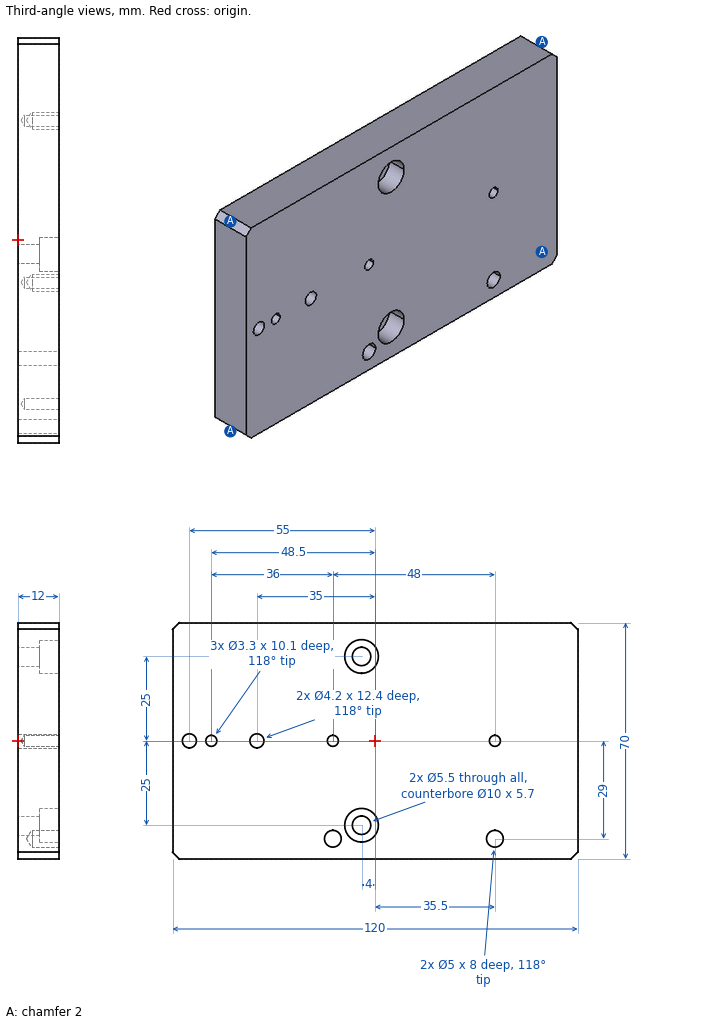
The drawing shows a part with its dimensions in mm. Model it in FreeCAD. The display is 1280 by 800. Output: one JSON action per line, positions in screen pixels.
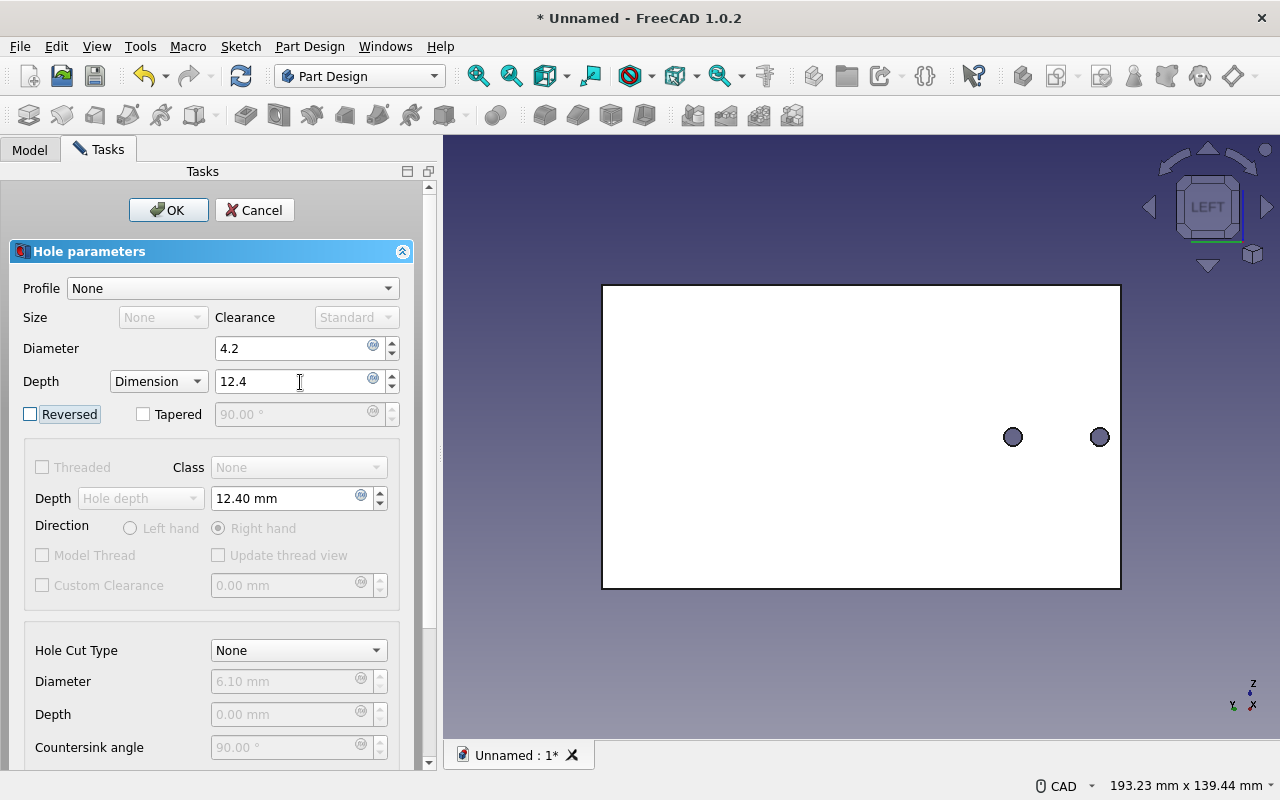
{"action": "left_click", "coordinate": [169, 210]}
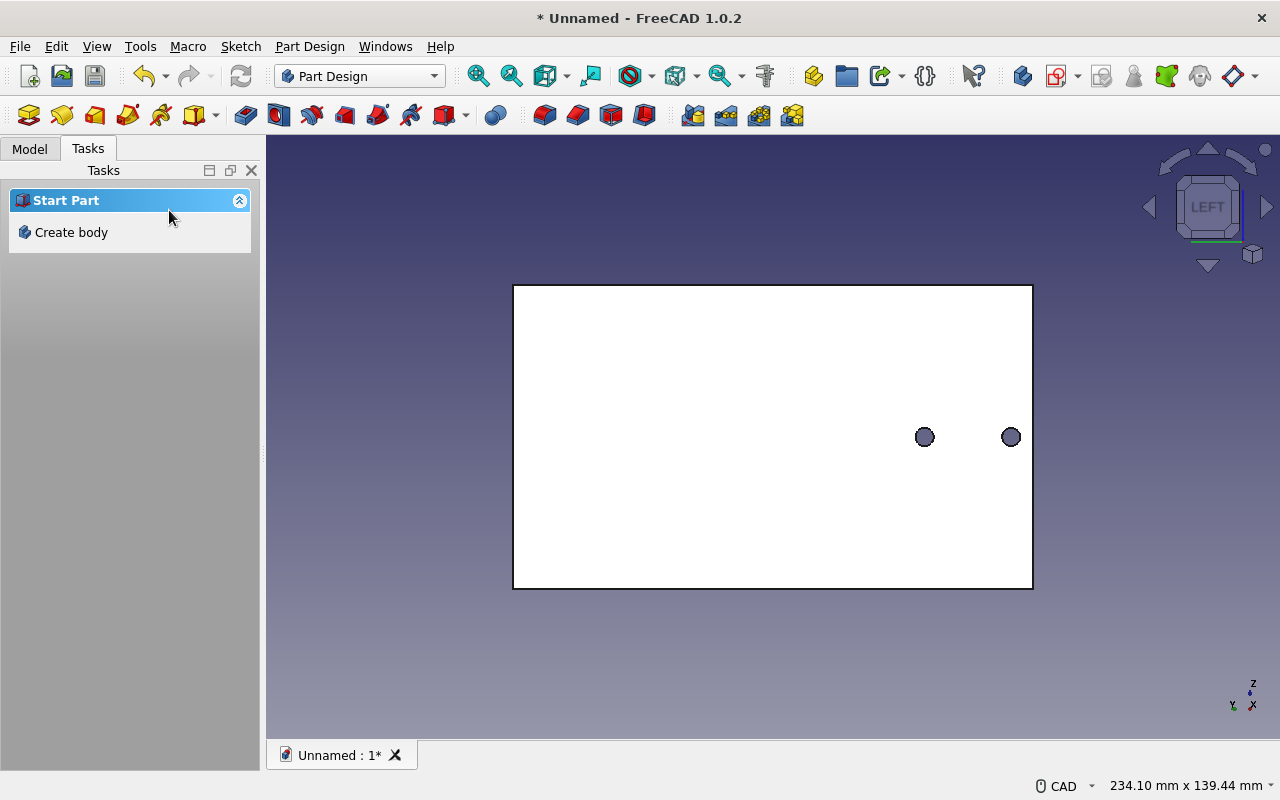
{"action": "key", "text": "0"}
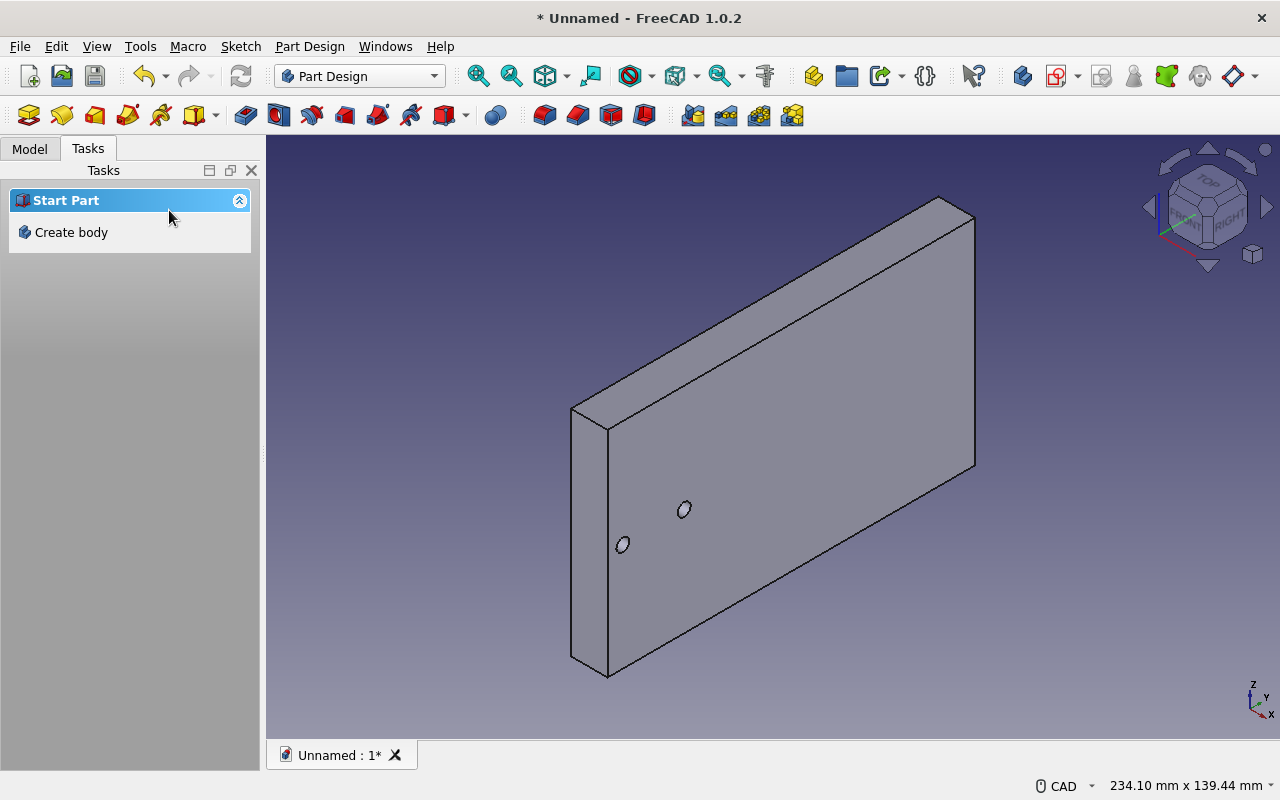
{"action": "left_click", "coordinate": [844, 416]}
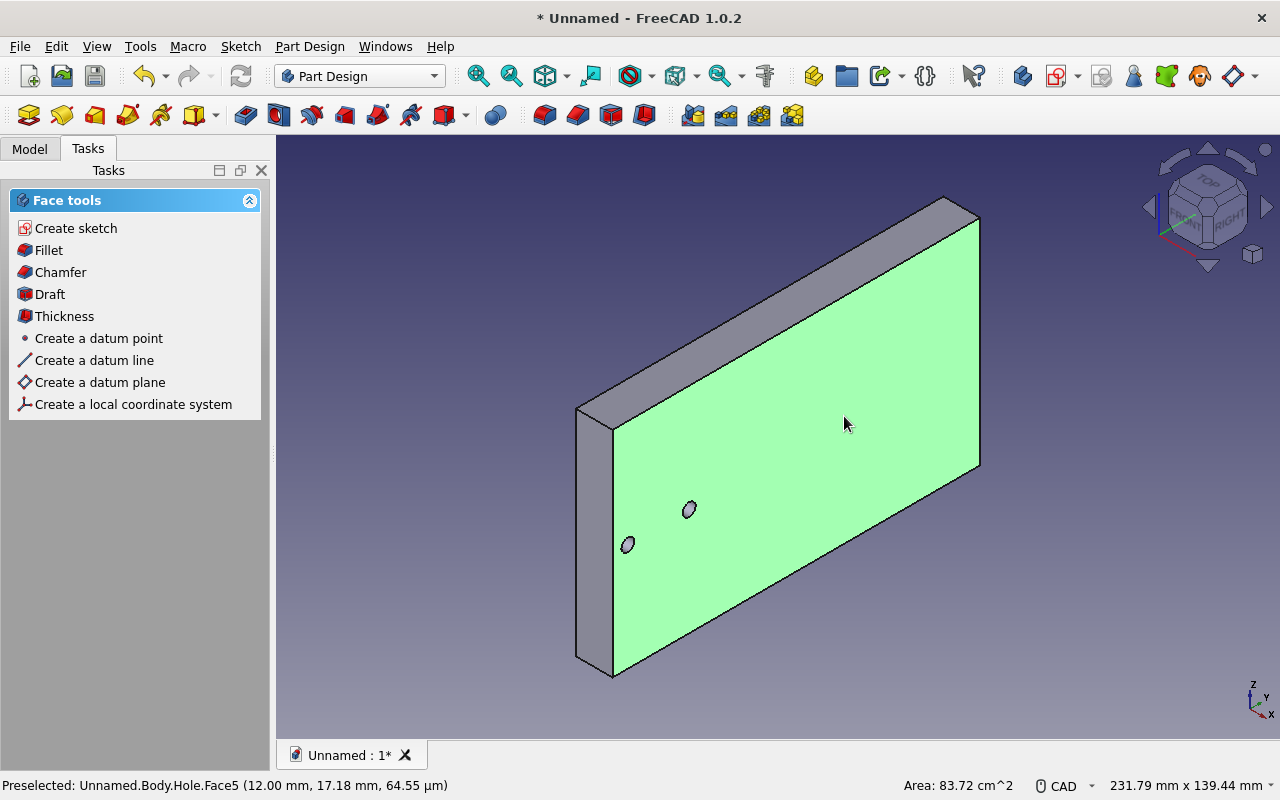
{"action": "left_click", "coordinate": [1056, 76]}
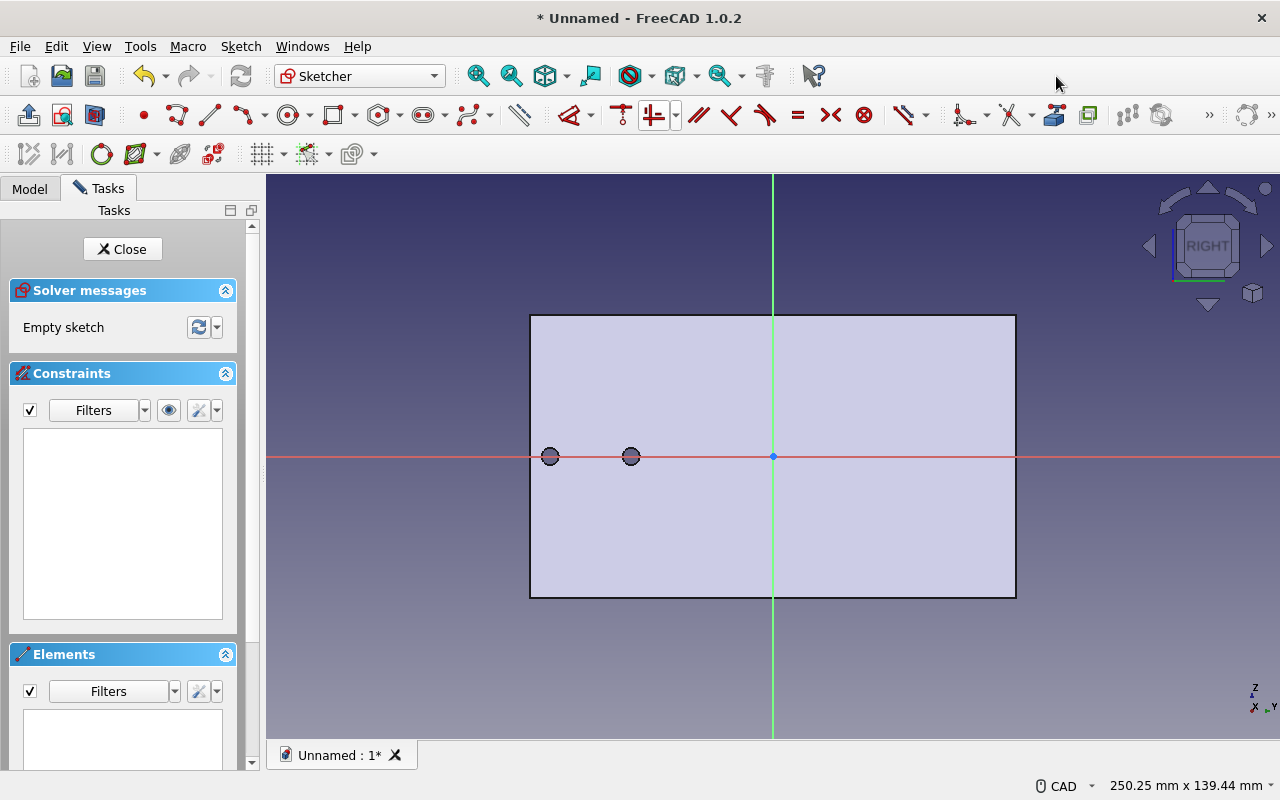
{"action": "scroll", "coordinate": [871, 457], "scroll_direction": "up", "scroll_amount": 2}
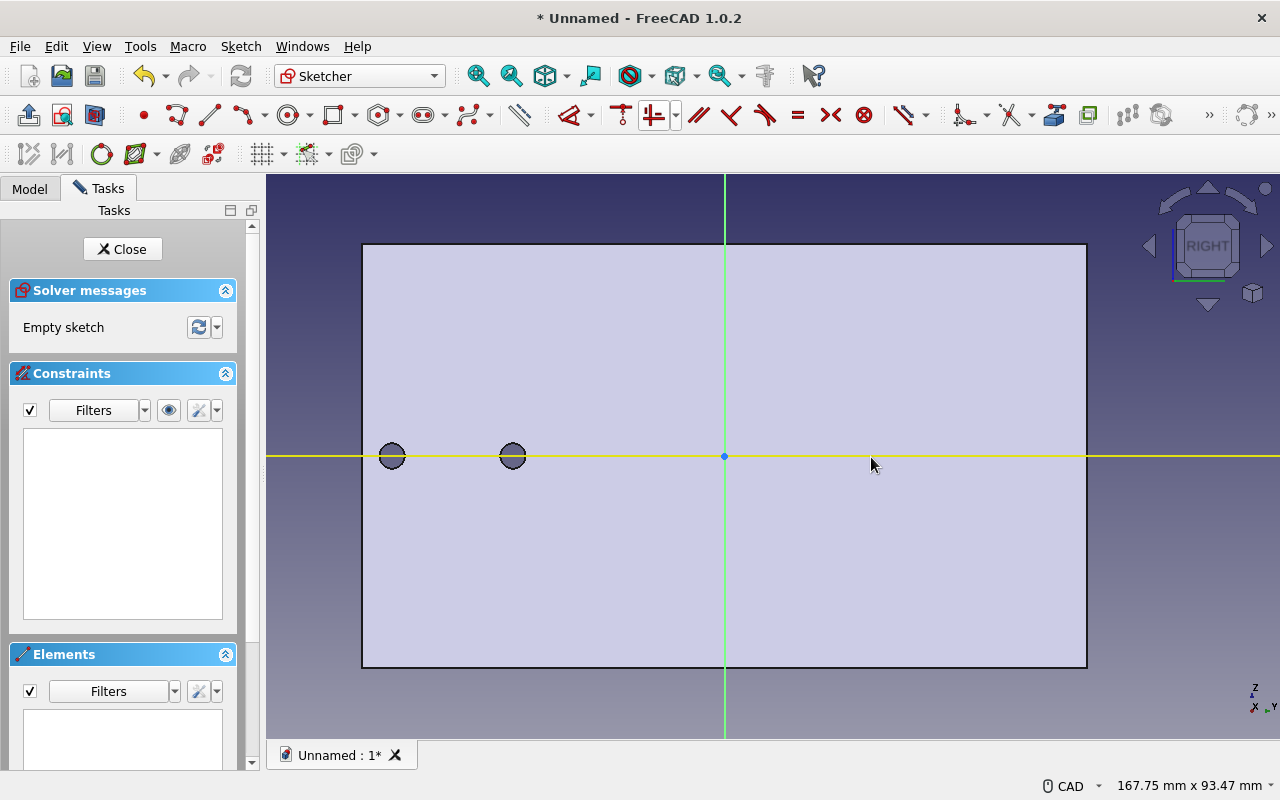
{"action": "left_click", "coordinate": [288, 116]}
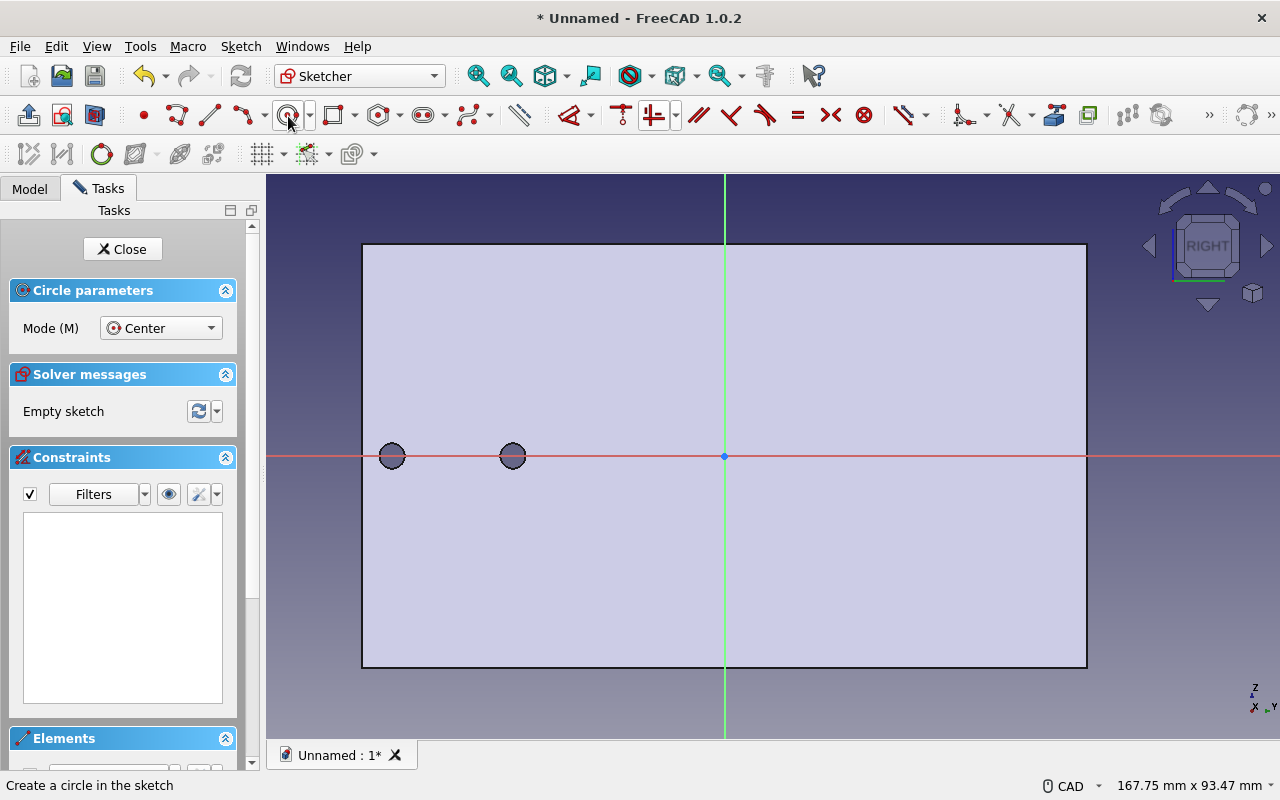
{"action": "scroll", "coordinate": [700, 607], "scroll_direction": "up", "scroll_amount": 2}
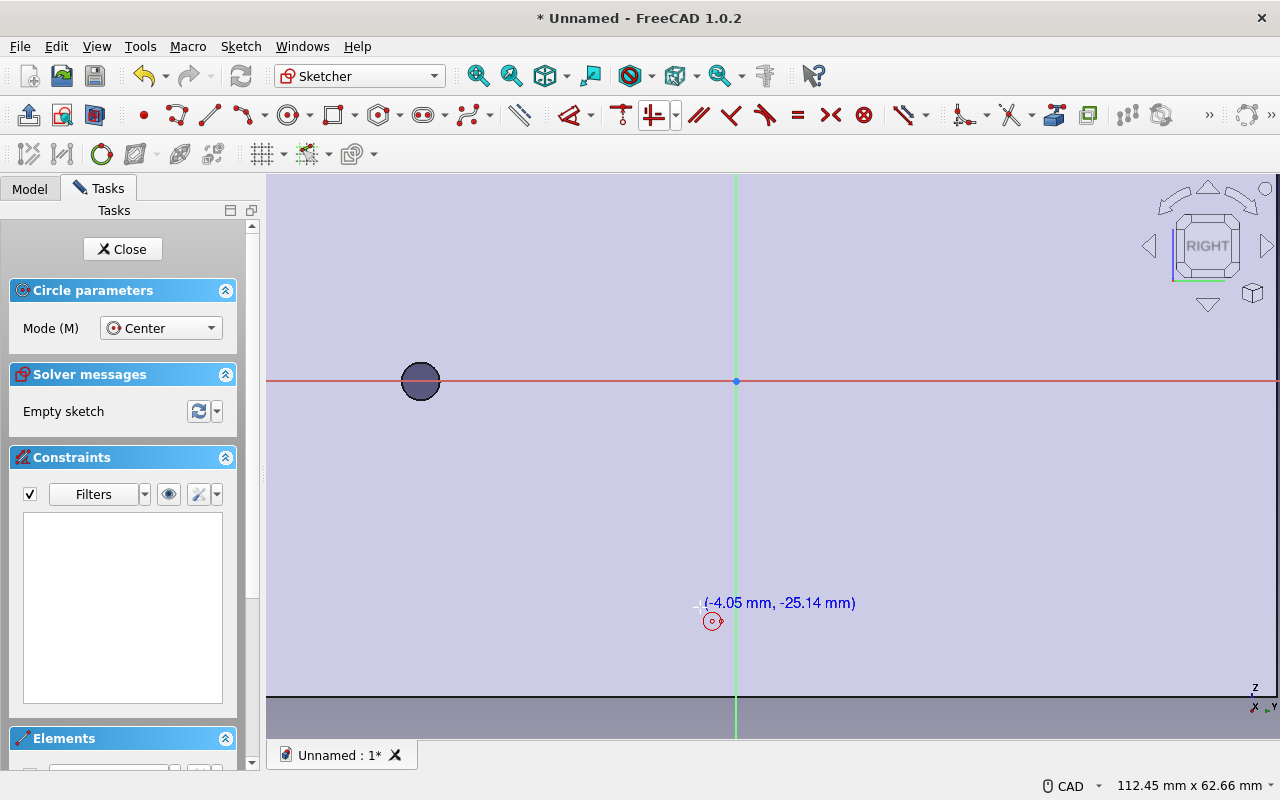
{"action": "left_click", "coordinate": [700, 607]}
{"action": "left_click", "coordinate": [718, 589]}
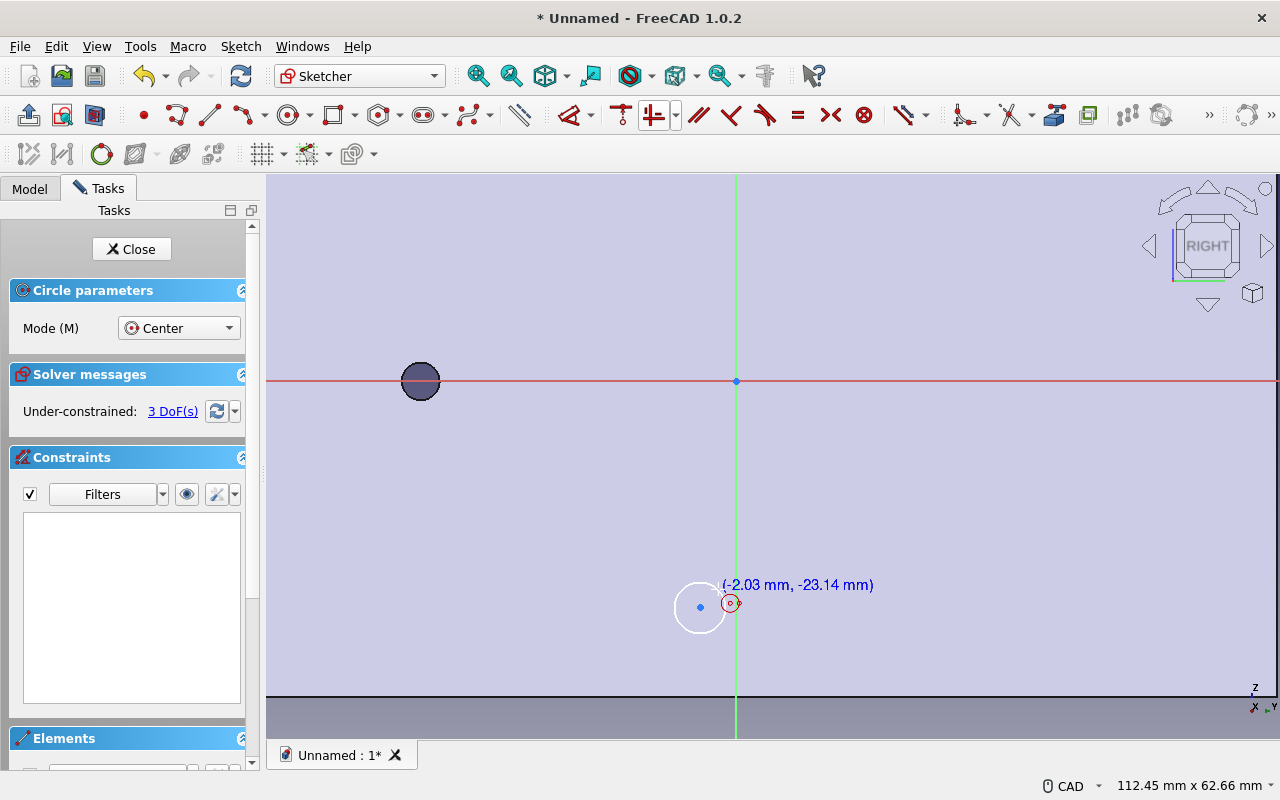
{"action": "scroll", "coordinate": [702, 609], "scroll_direction": "down", "scroll_amount": 2}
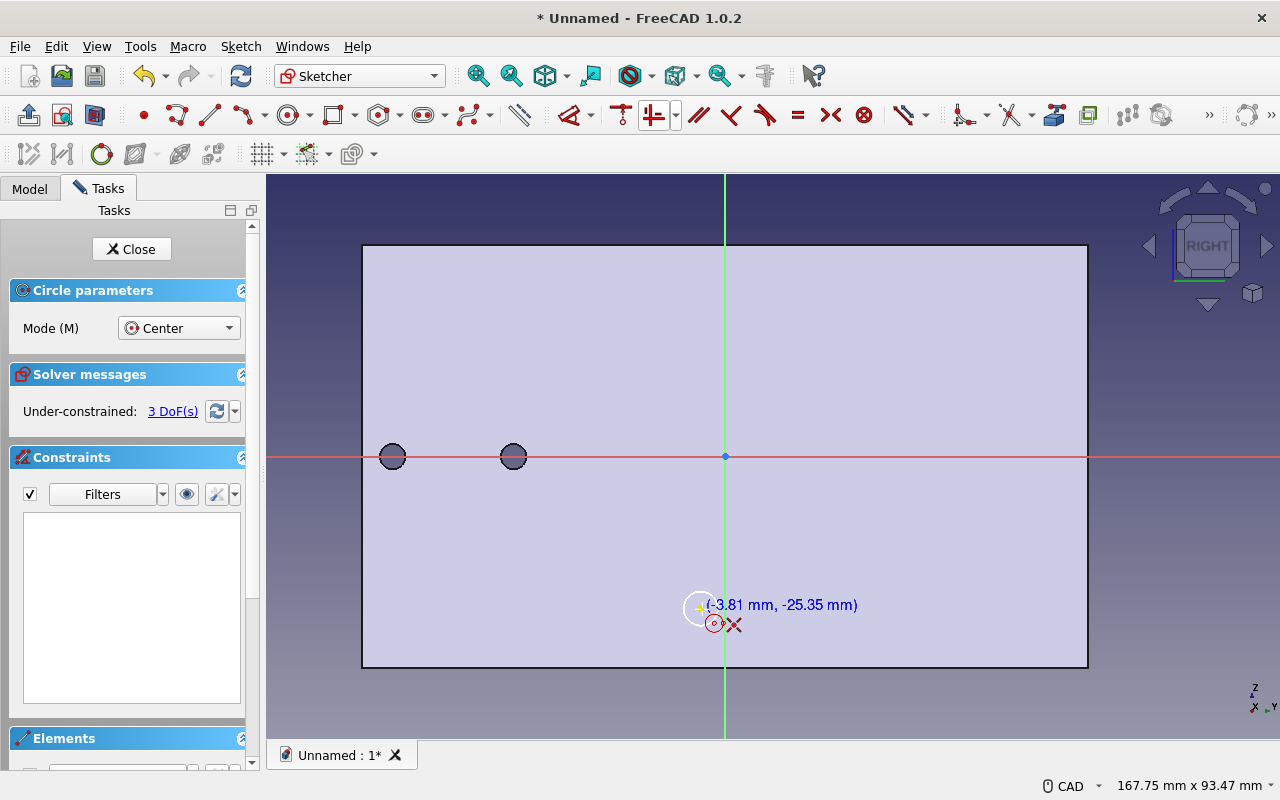
{"action": "scroll", "coordinate": [701, 306], "scroll_direction": "up", "scroll_amount": 2}